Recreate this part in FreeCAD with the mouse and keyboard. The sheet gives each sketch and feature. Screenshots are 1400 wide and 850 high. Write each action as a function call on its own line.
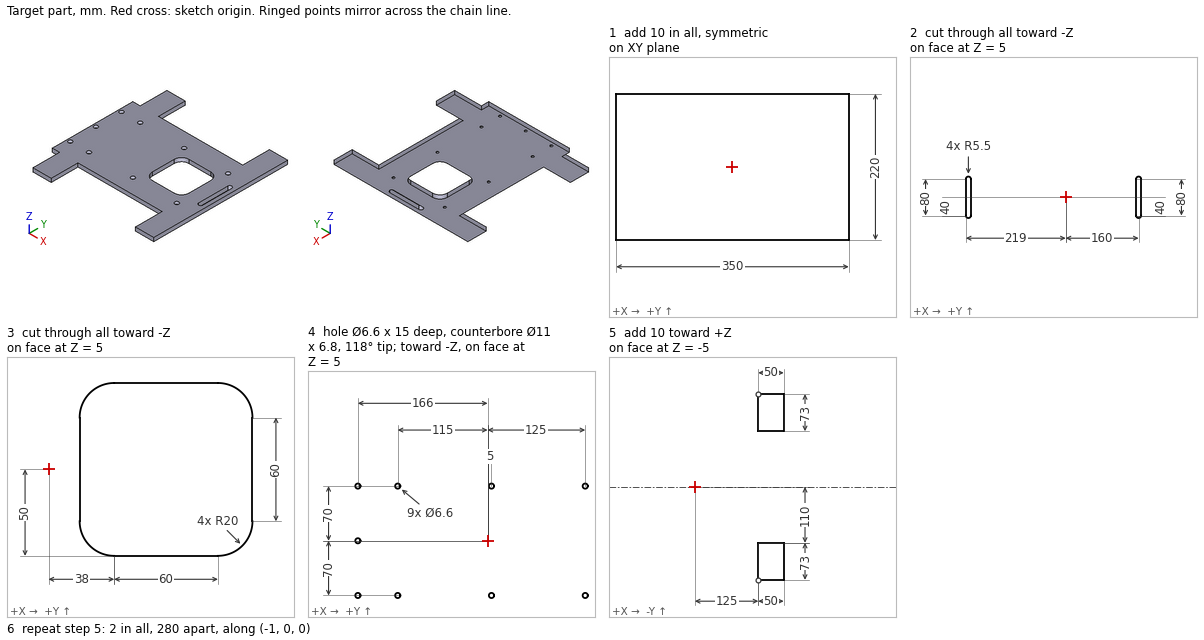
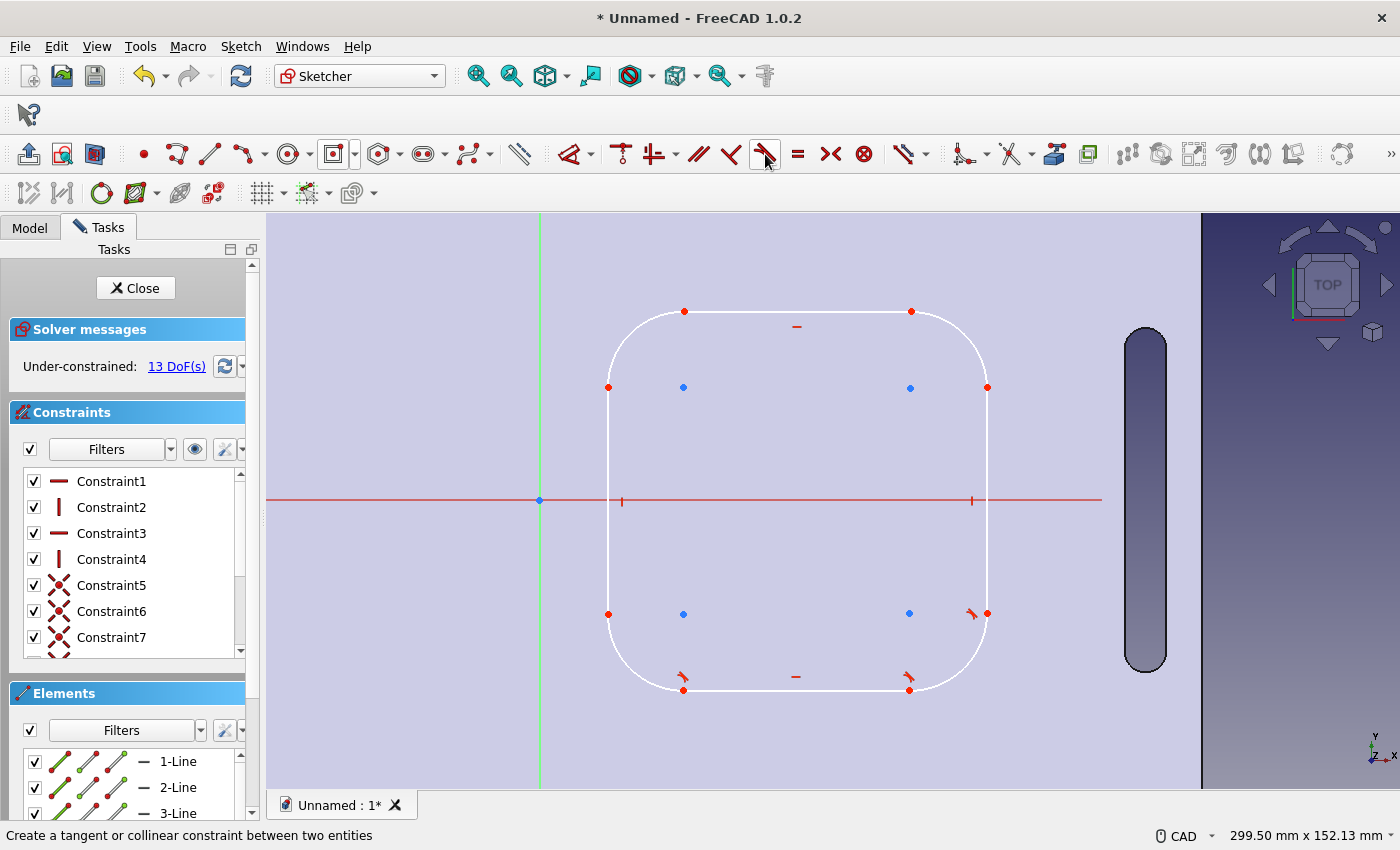
click(987, 546)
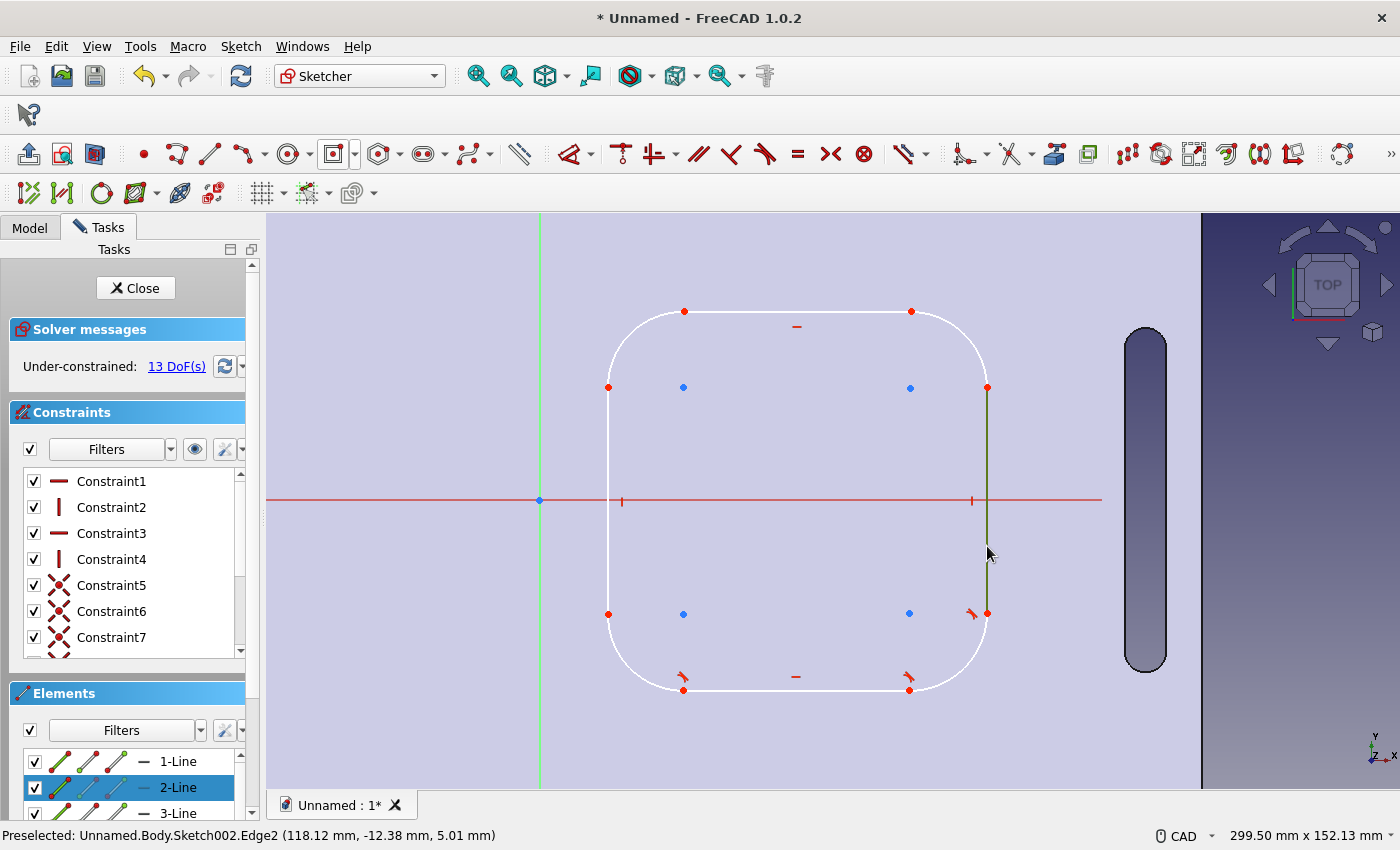
click(978, 354)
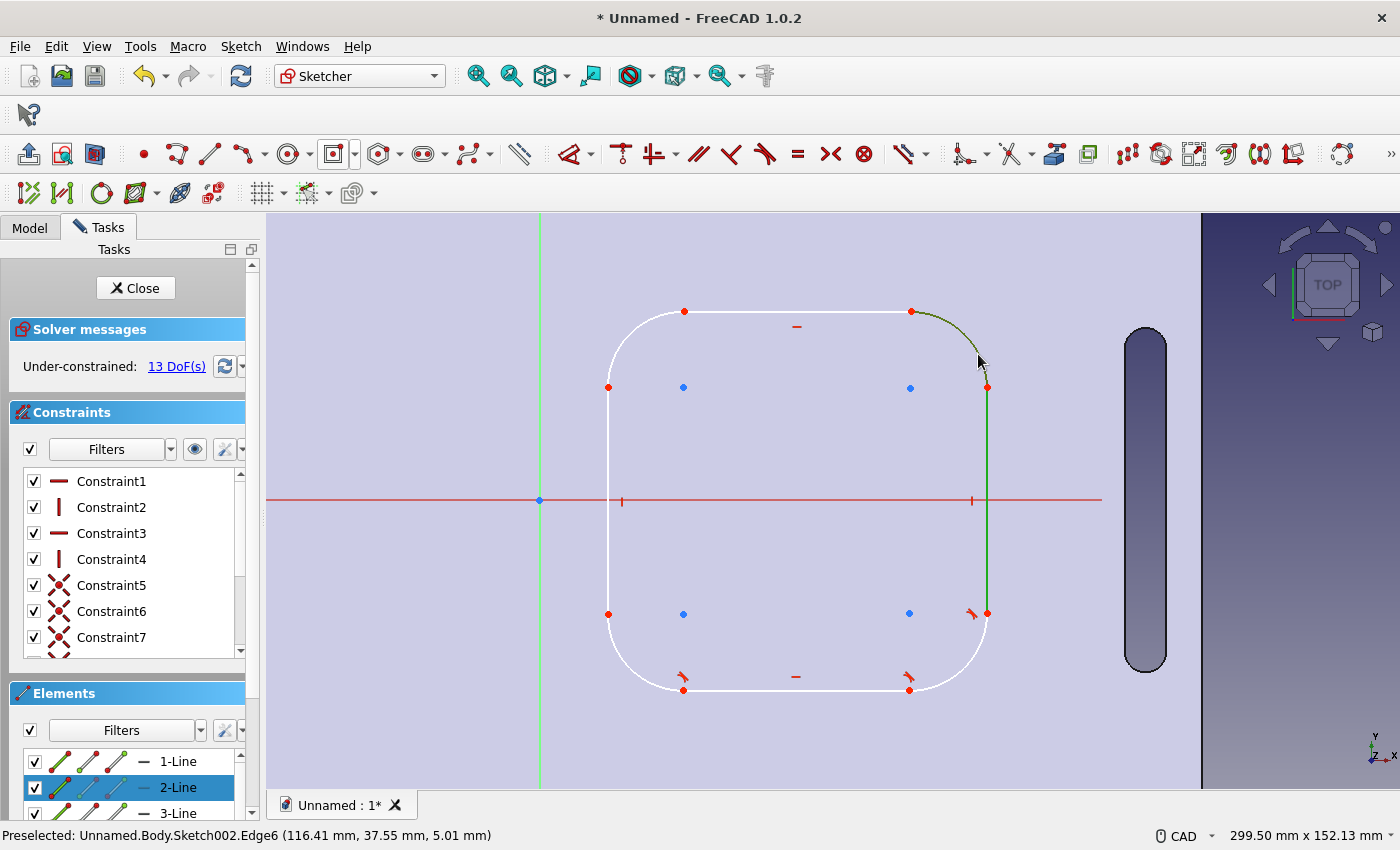
click(765, 154)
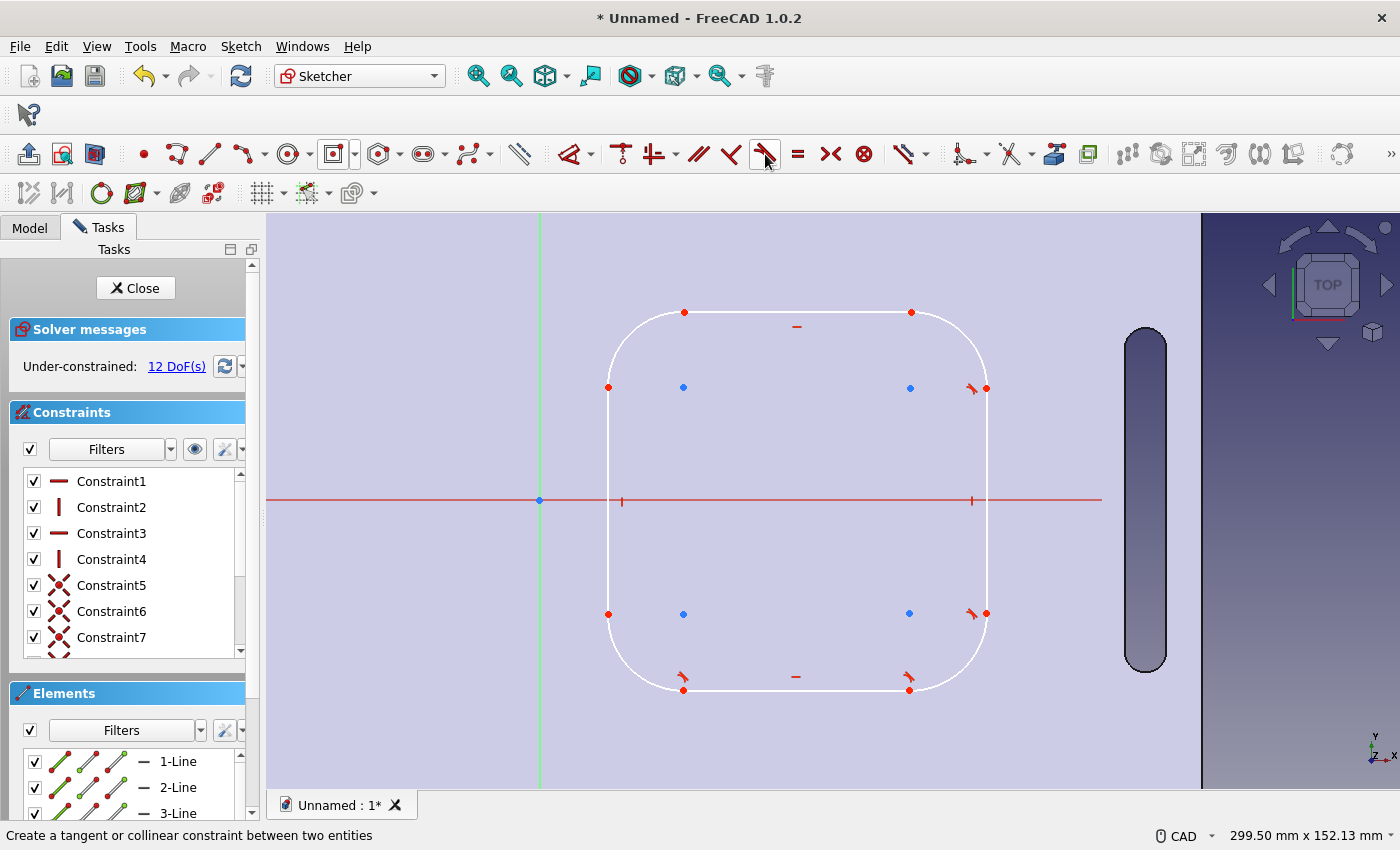
click(843, 312)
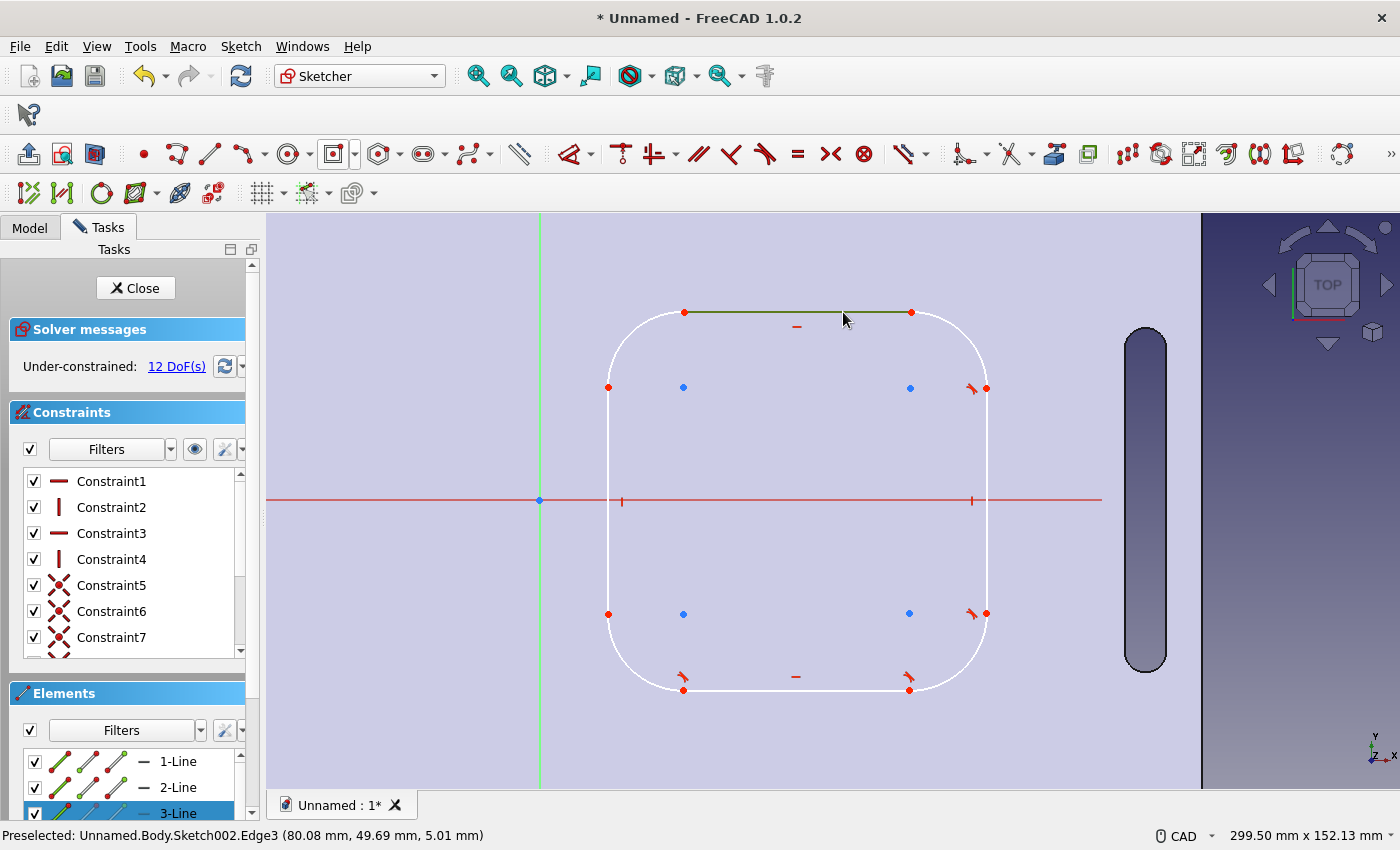
click(979, 354)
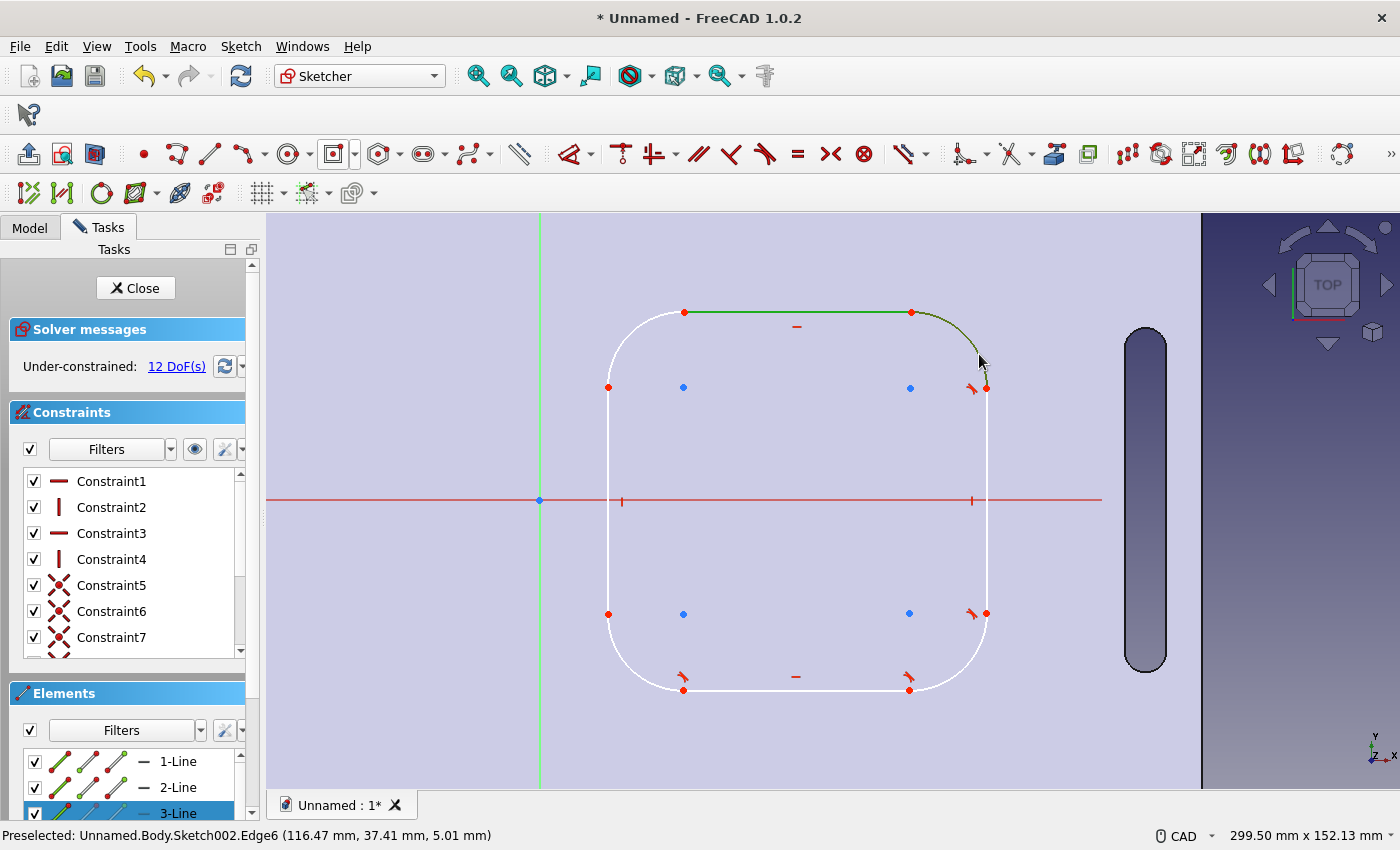
click(765, 154)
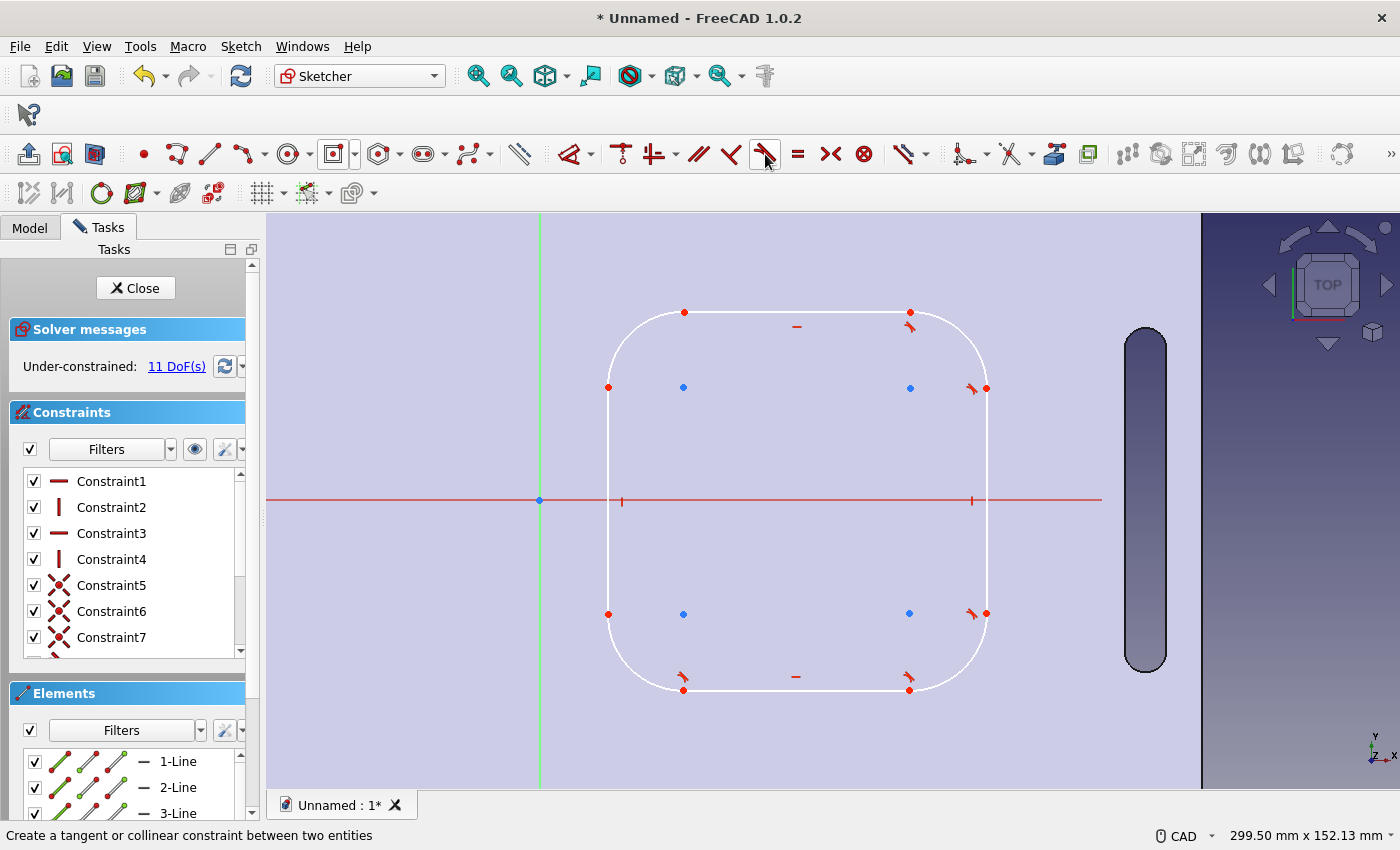
click(842, 312)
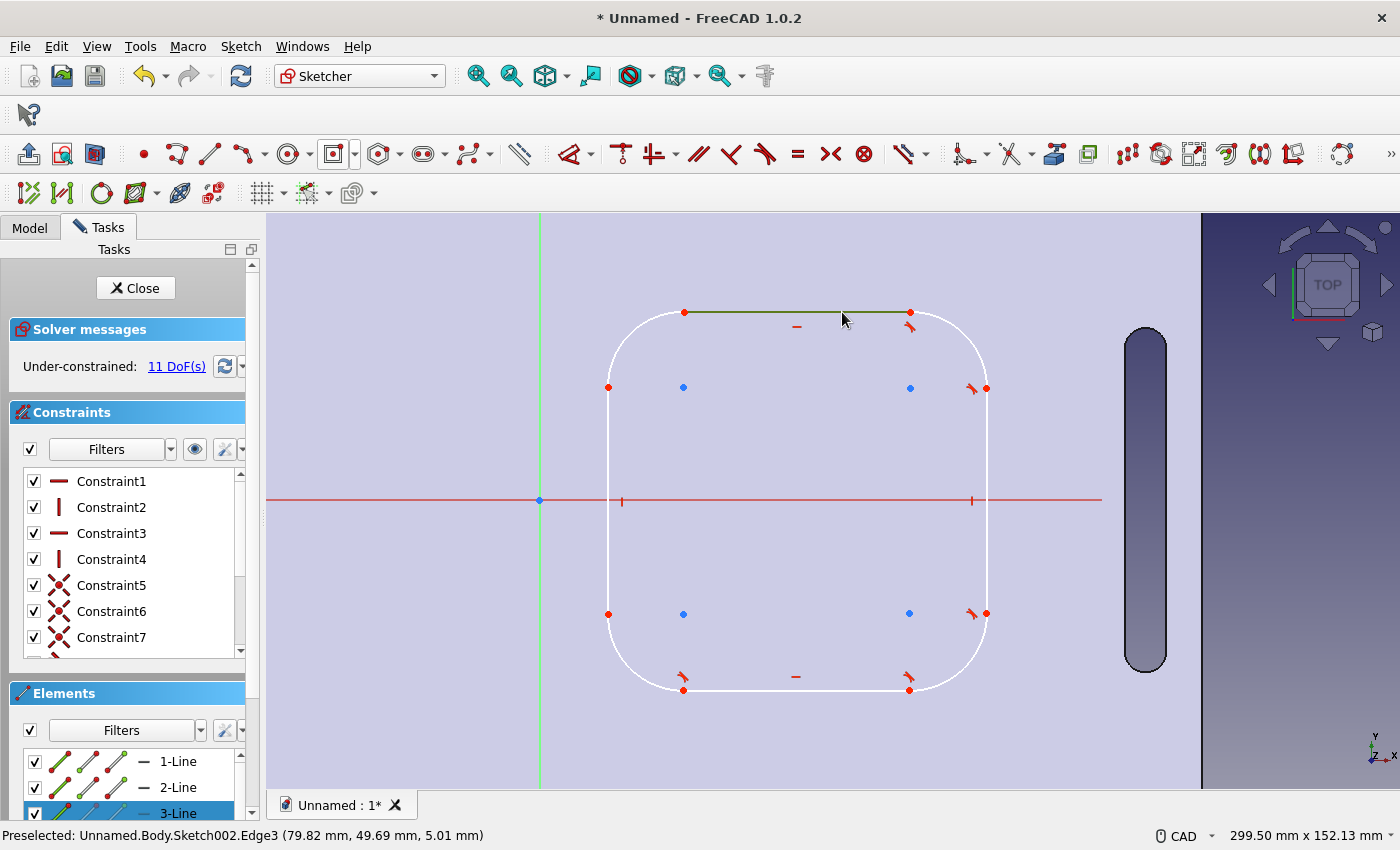
click(649, 320)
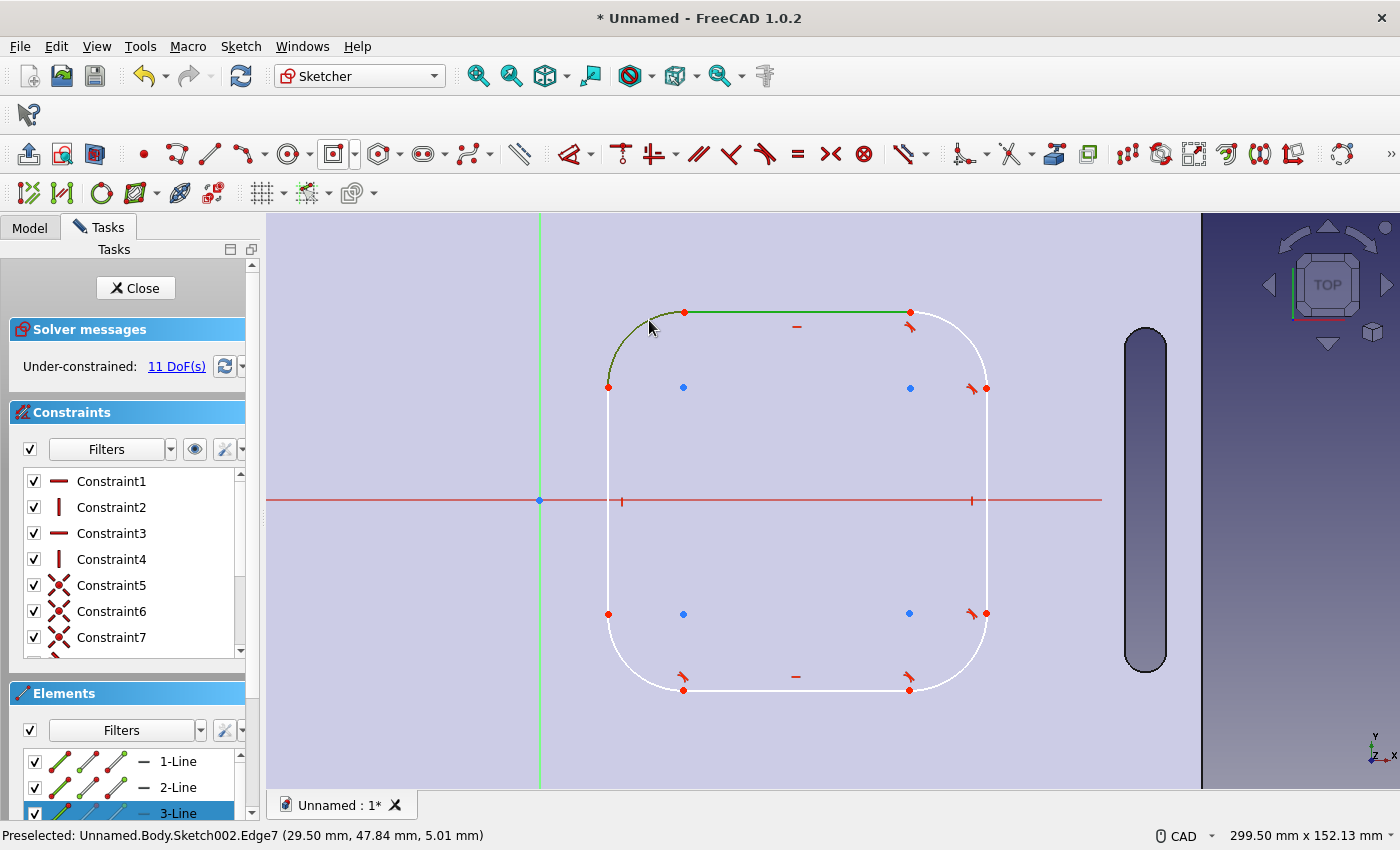
key(t)